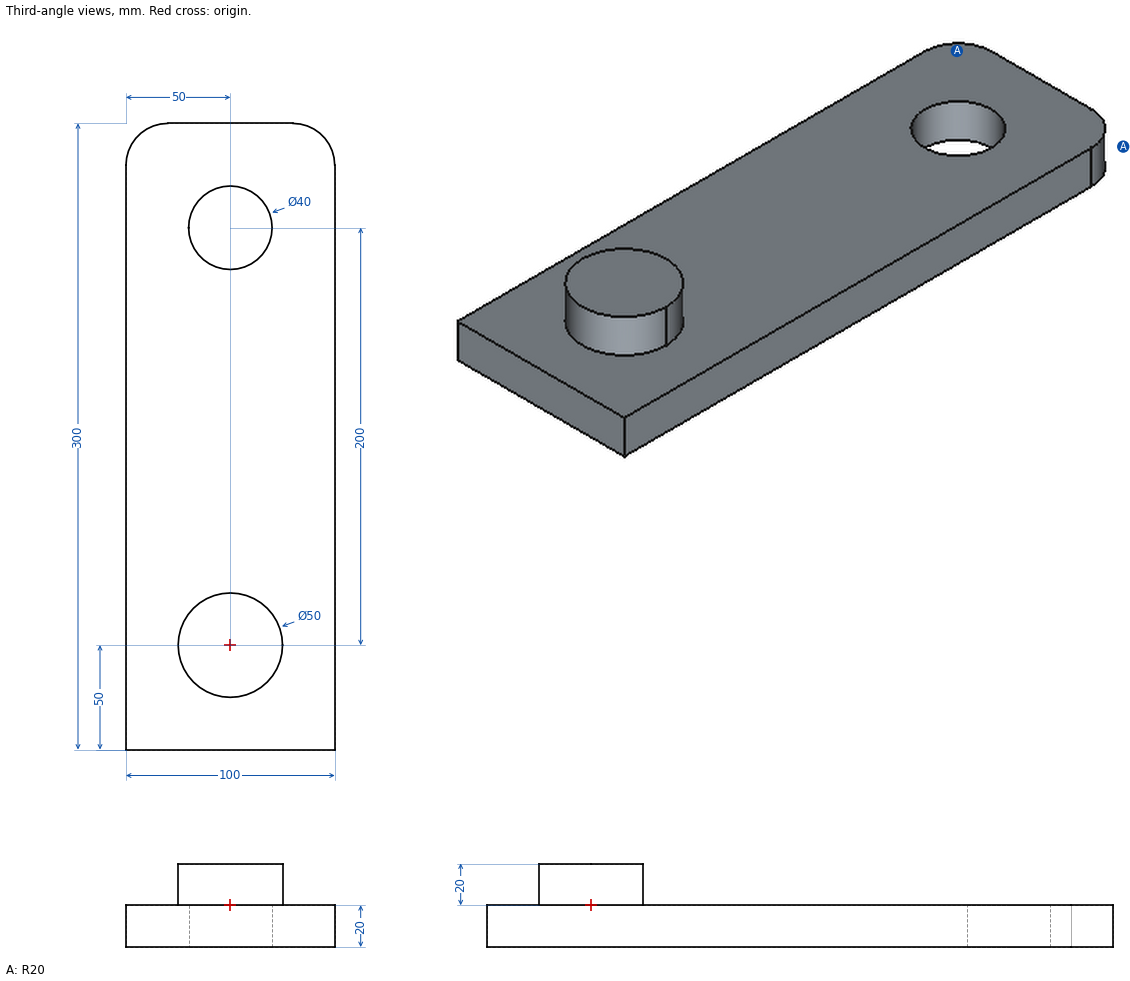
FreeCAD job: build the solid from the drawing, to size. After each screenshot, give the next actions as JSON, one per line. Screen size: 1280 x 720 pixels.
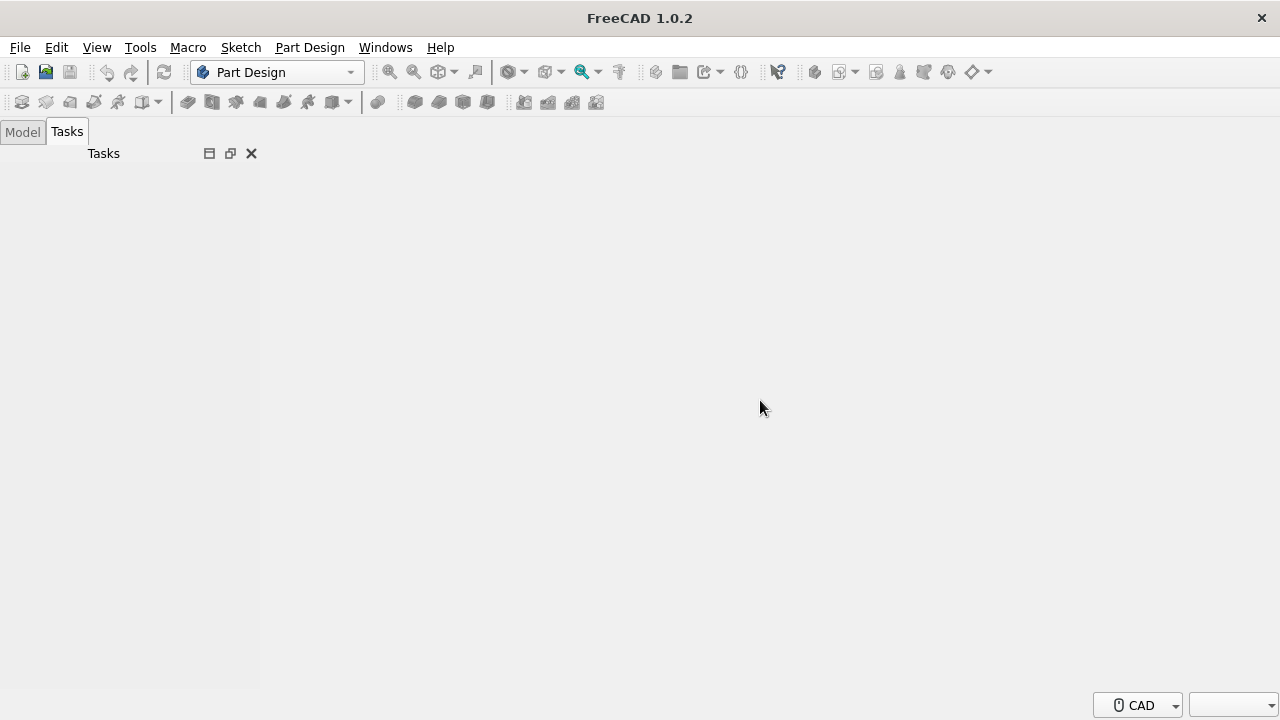
{"action": "left_click", "coordinate": [22, 72]}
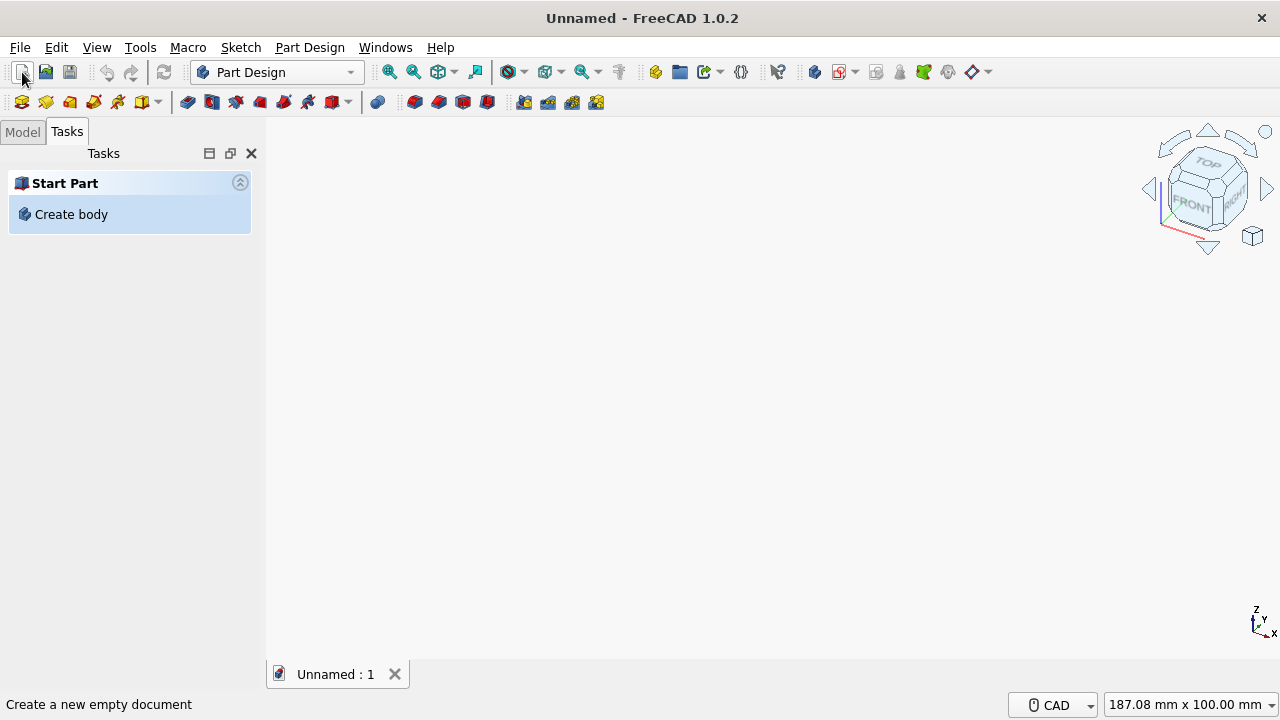
{"action": "left_click", "coordinate": [840, 72]}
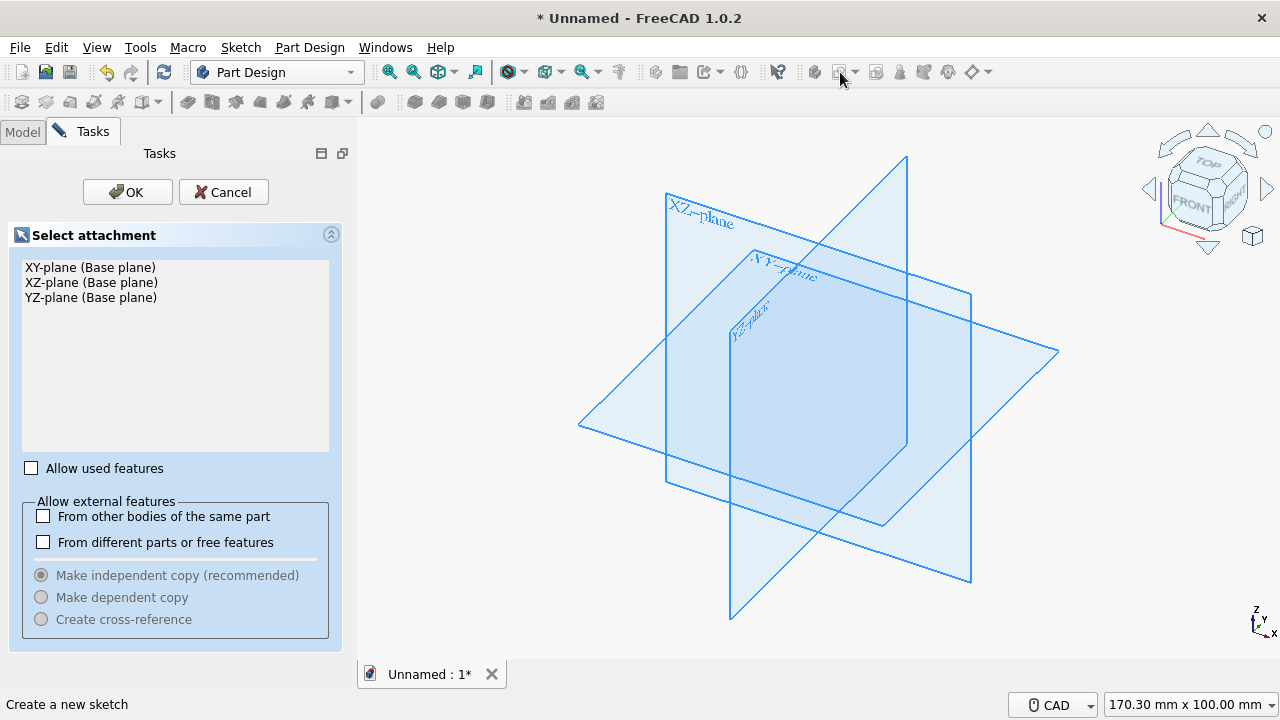
{"action": "left_click", "coordinate": [82, 268]}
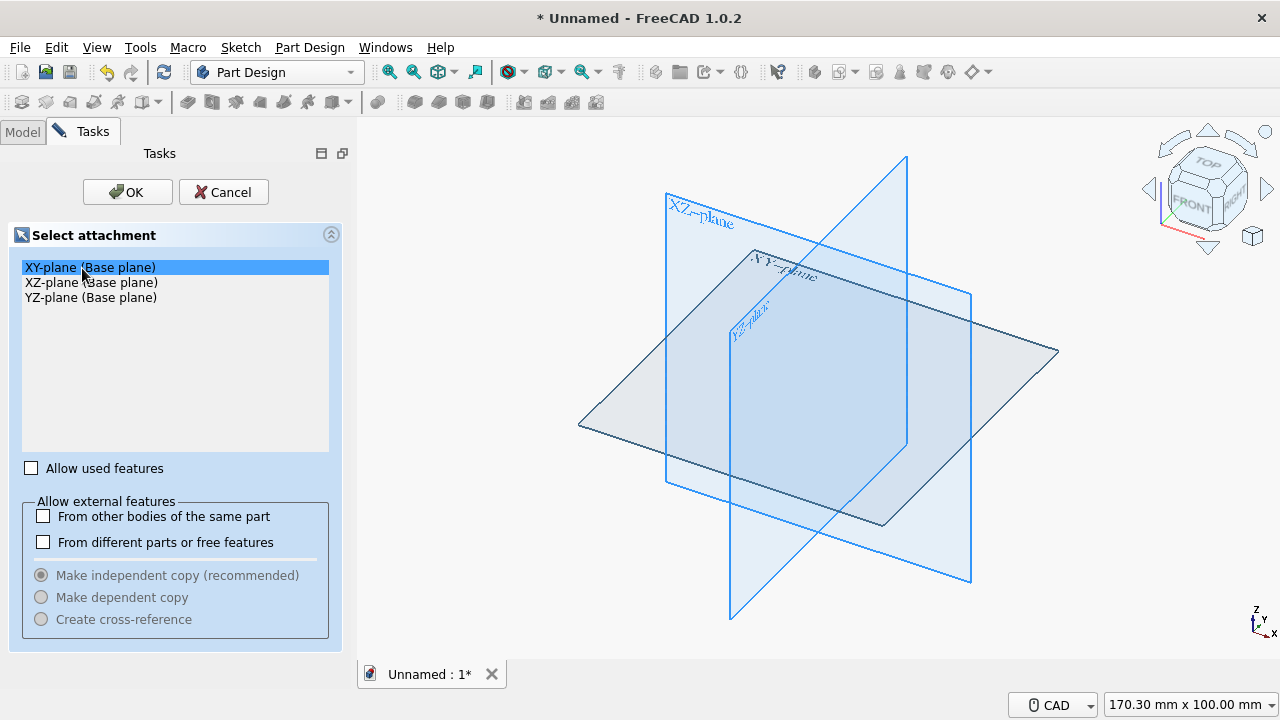
{"action": "left_click", "coordinate": [128, 192]}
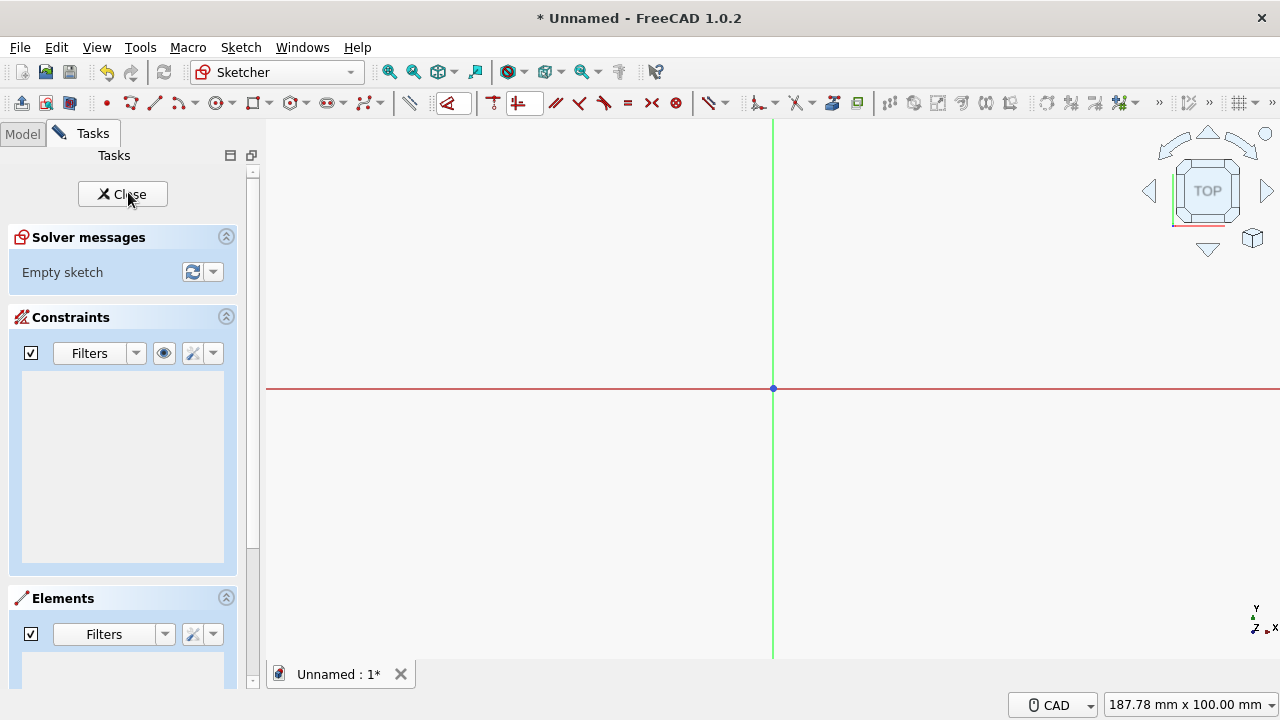
{"action": "left_click", "coordinate": [216, 104]}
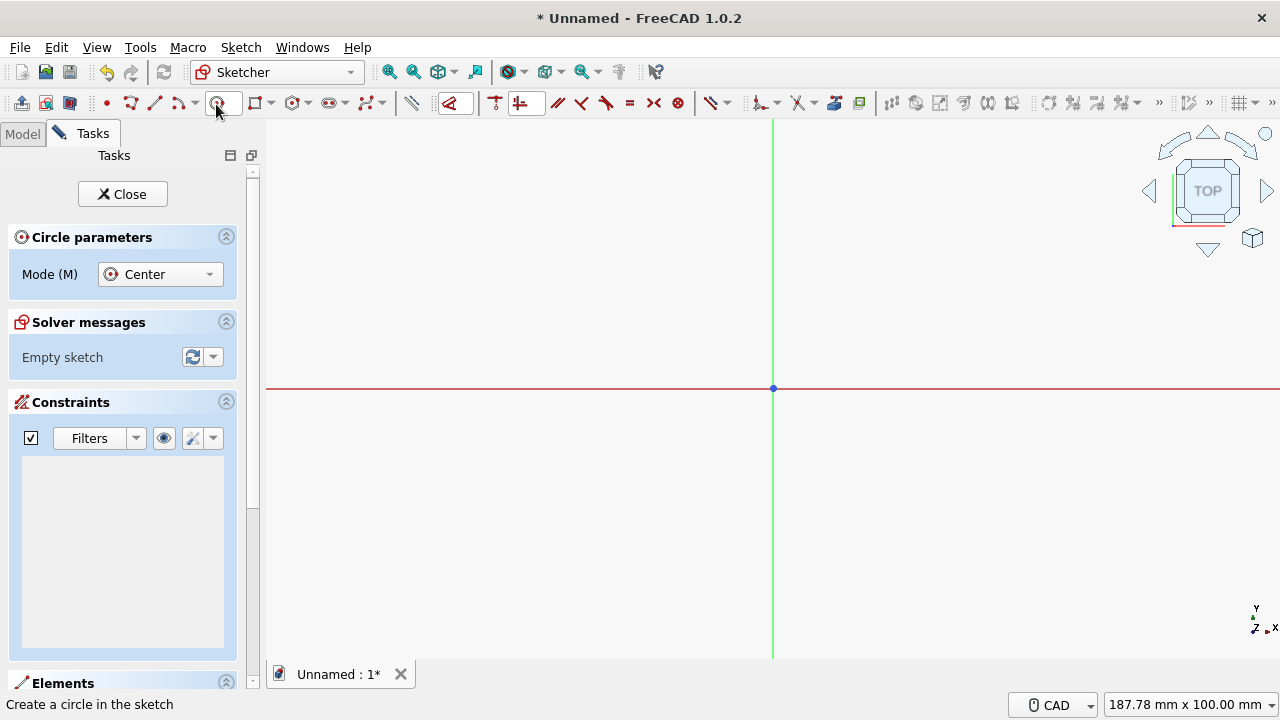
{"action": "left_click", "coordinate": [773, 389]}
{"action": "left_click", "coordinate": [868, 294]}
{"action": "key", "text": "Escape"}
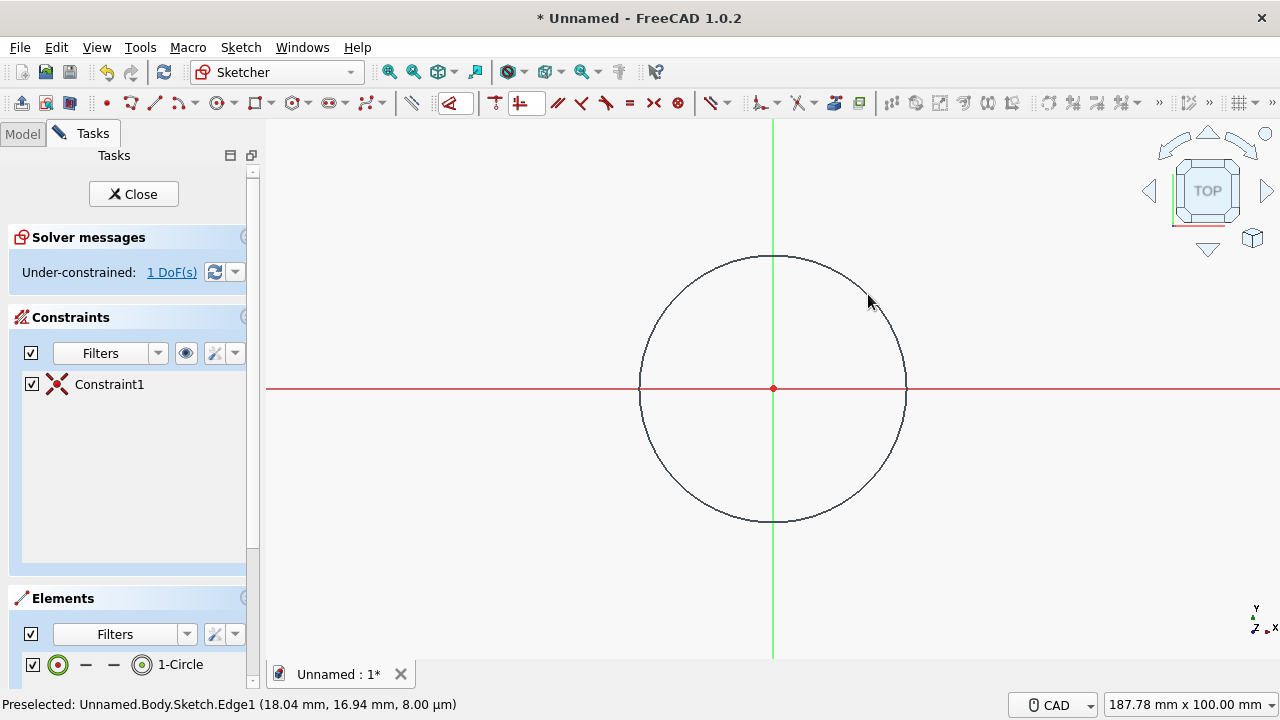
{"action": "left_click", "coordinate": [867, 294]}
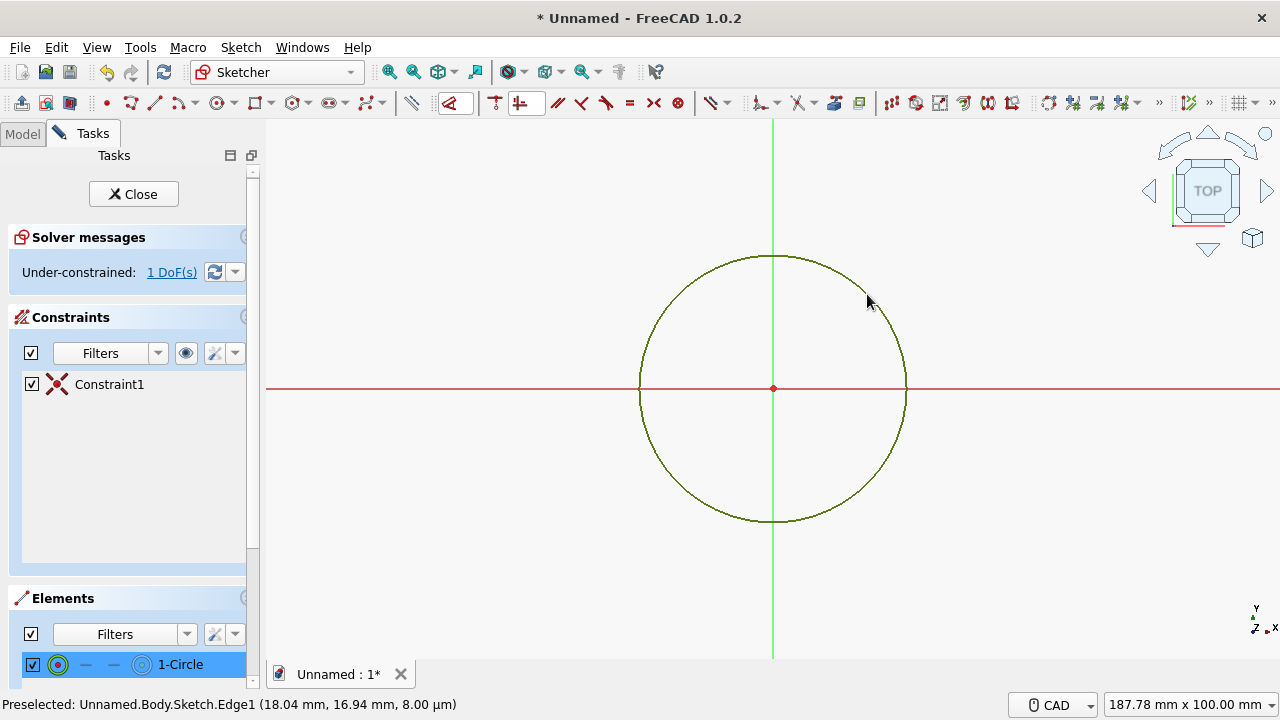
{"action": "left_click", "coordinate": [468, 104]}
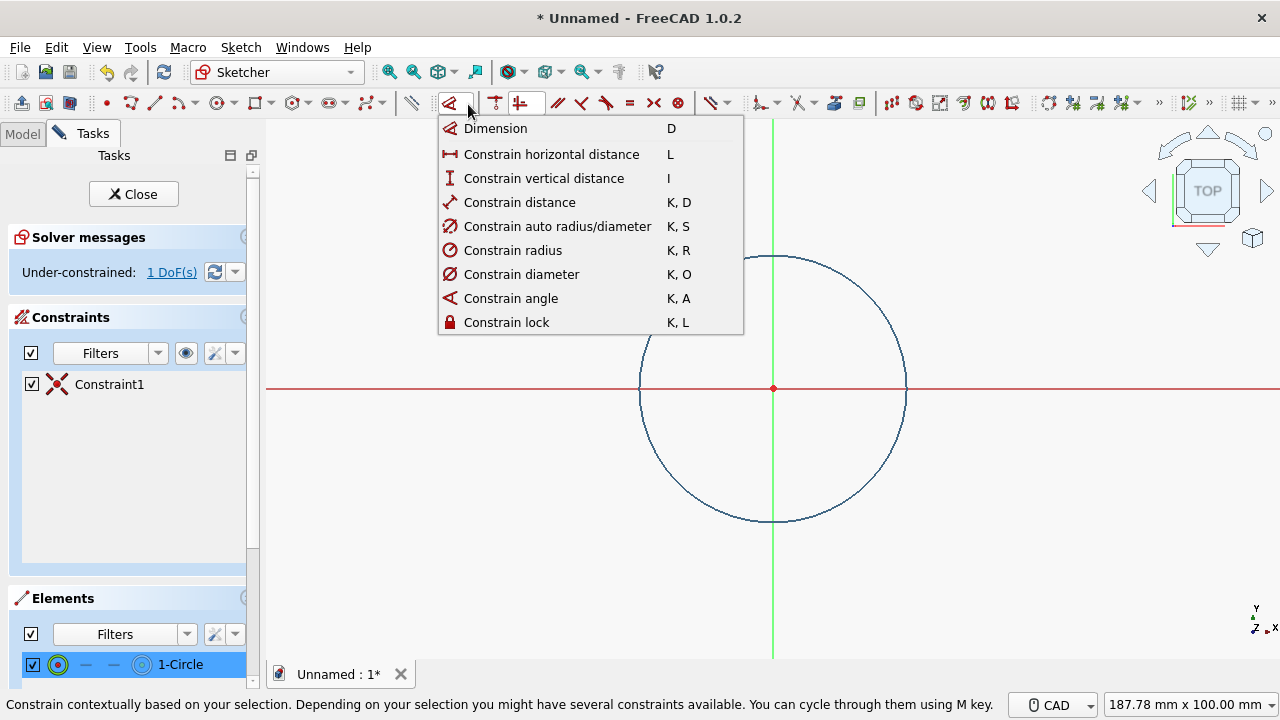
{"action": "left_click", "coordinate": [591, 274]}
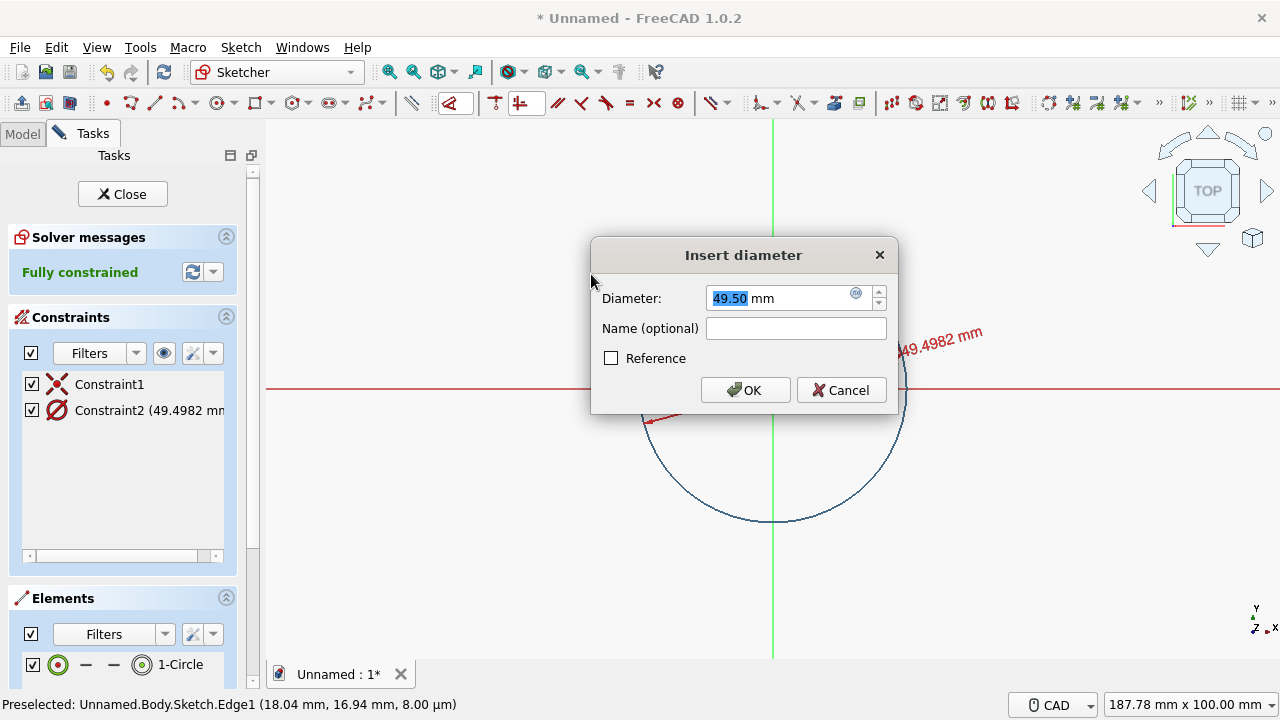
{"action": "type", "text": "50"}
{"action": "key", "text": "Return"}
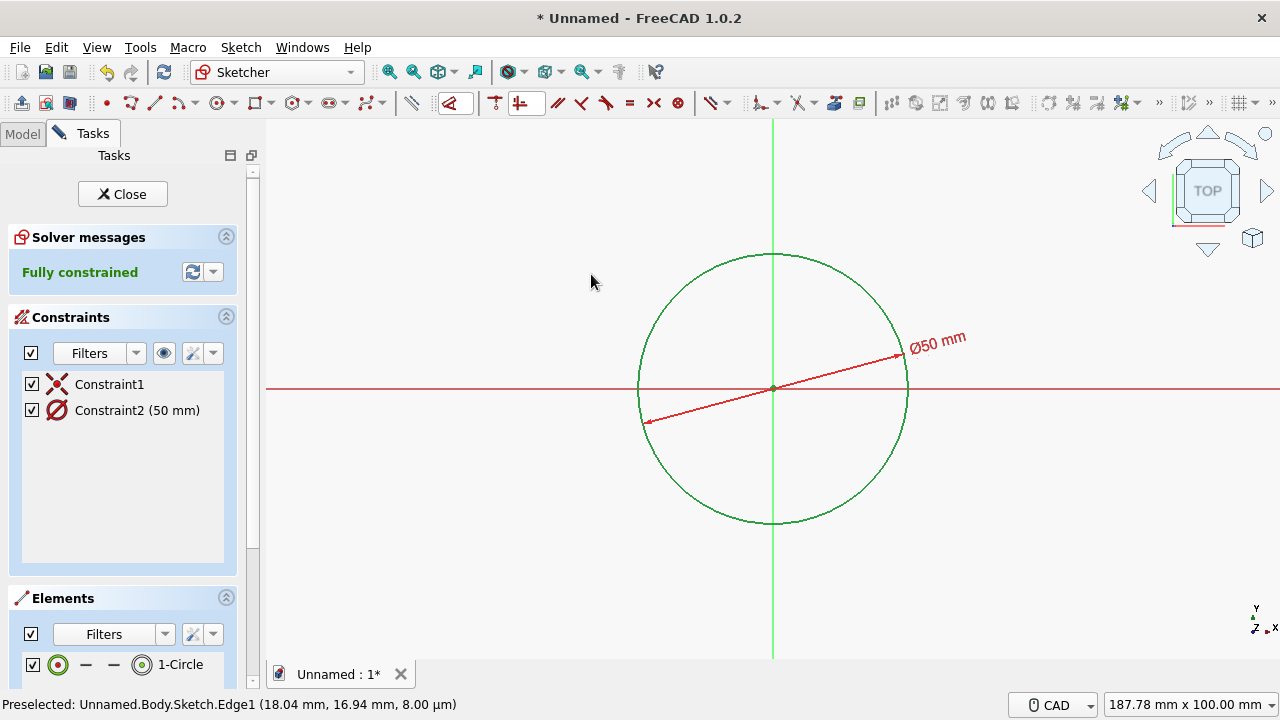
{"action": "left_click", "coordinate": [123, 194]}